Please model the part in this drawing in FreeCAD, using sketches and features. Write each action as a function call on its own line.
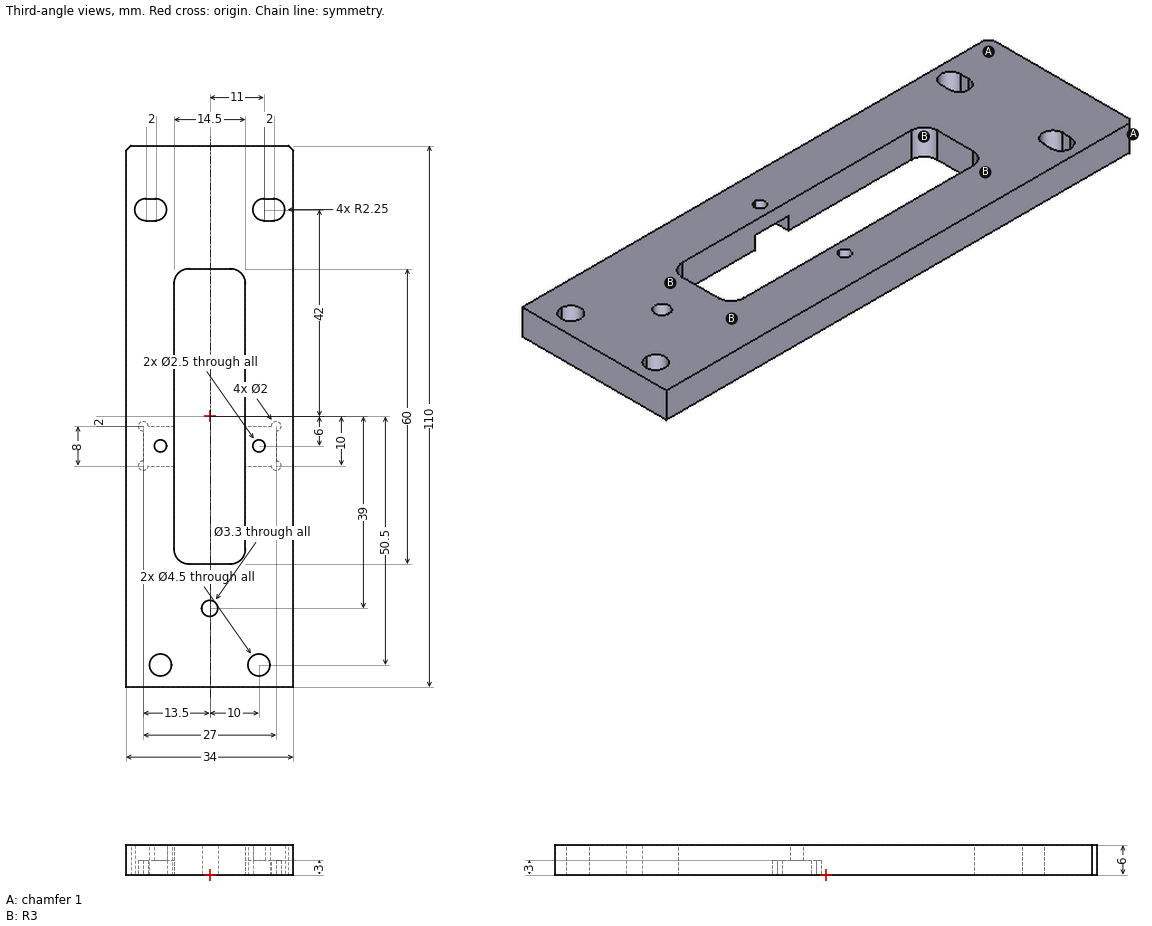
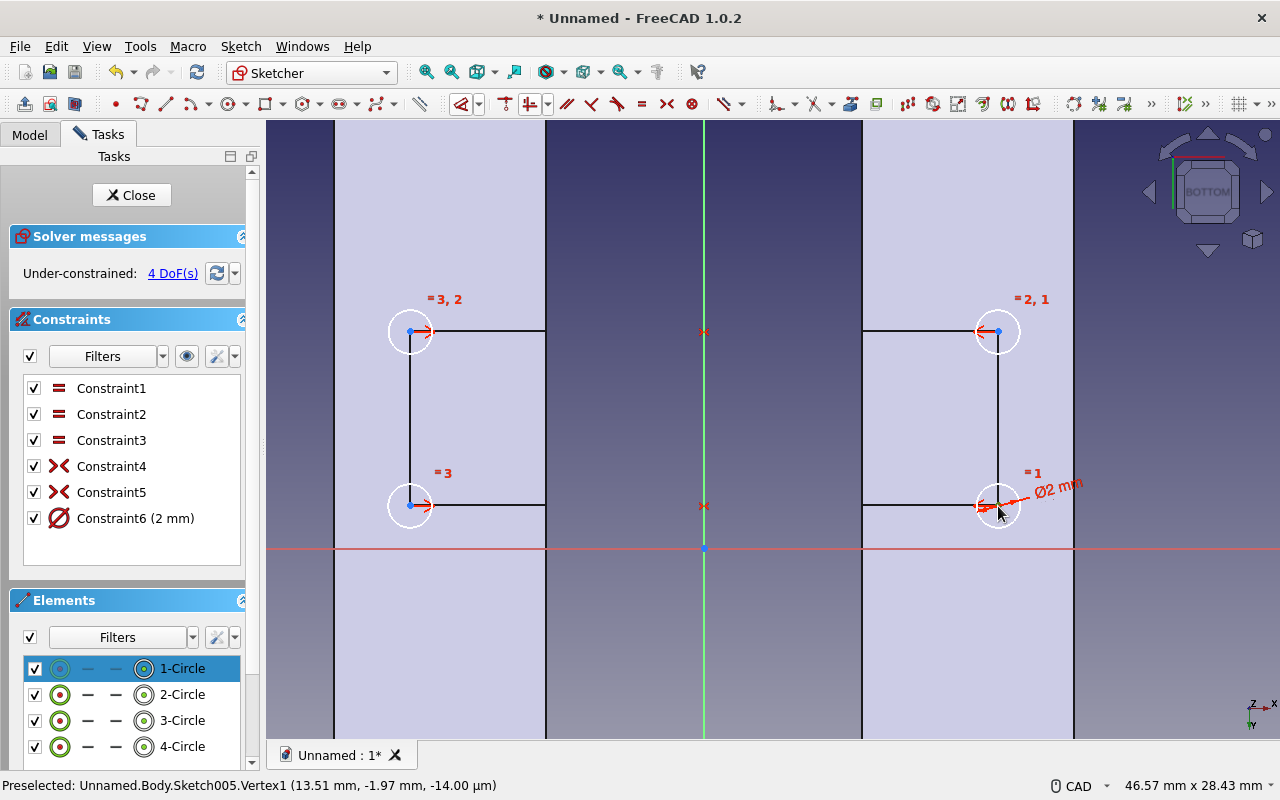
key(i)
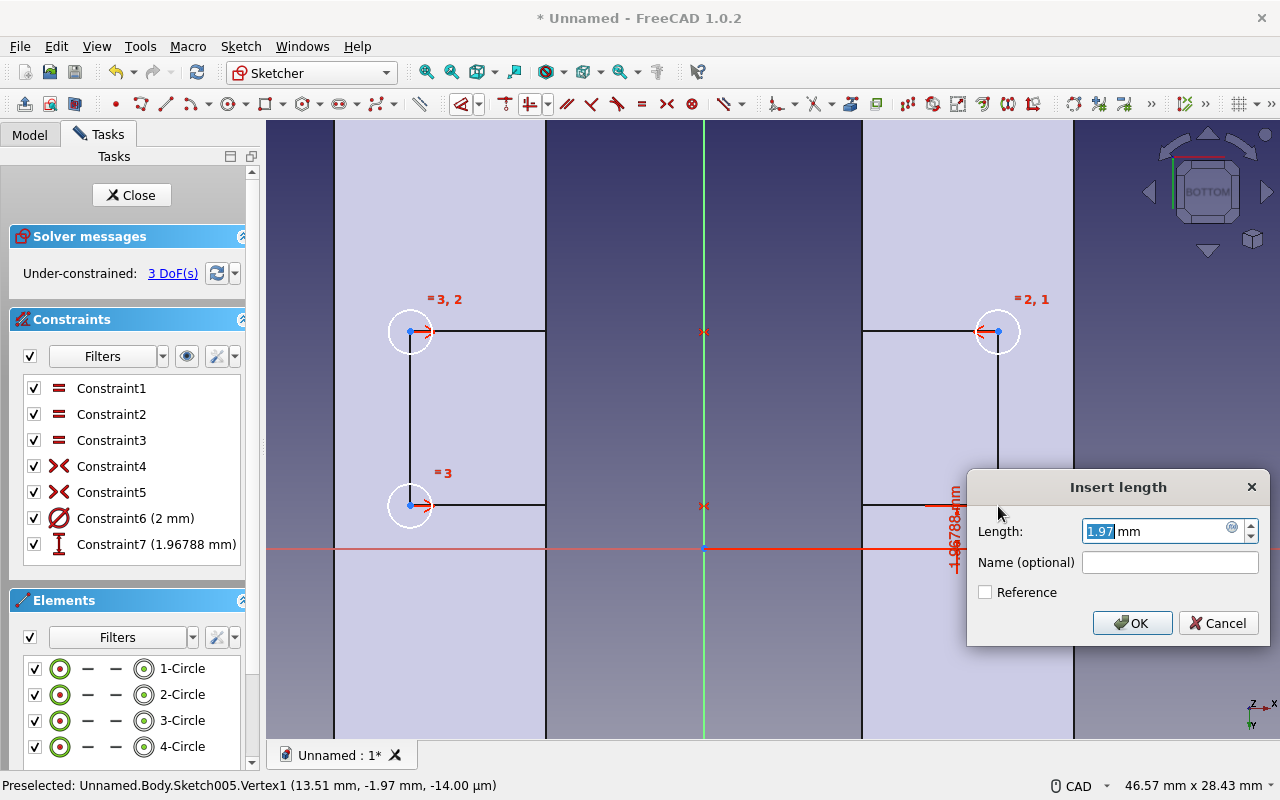
text(2)
key(Return)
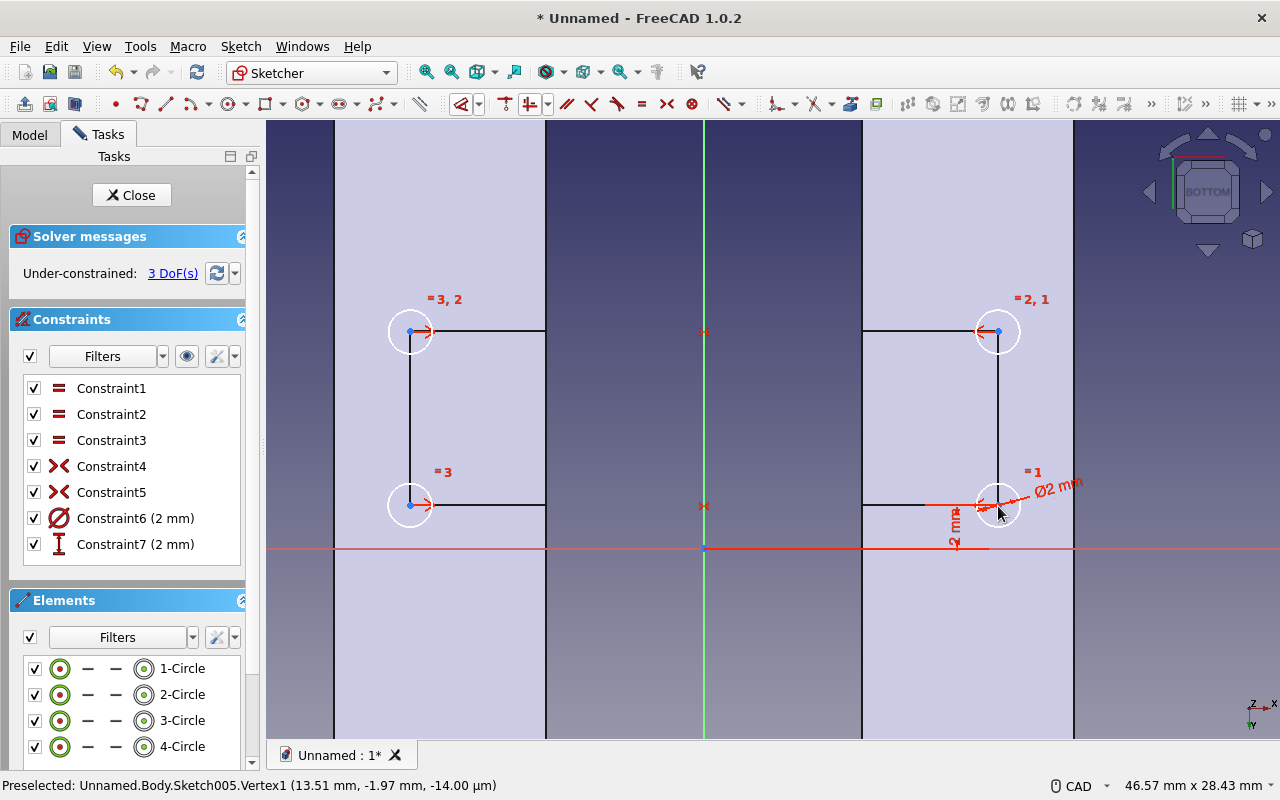
click(998, 332)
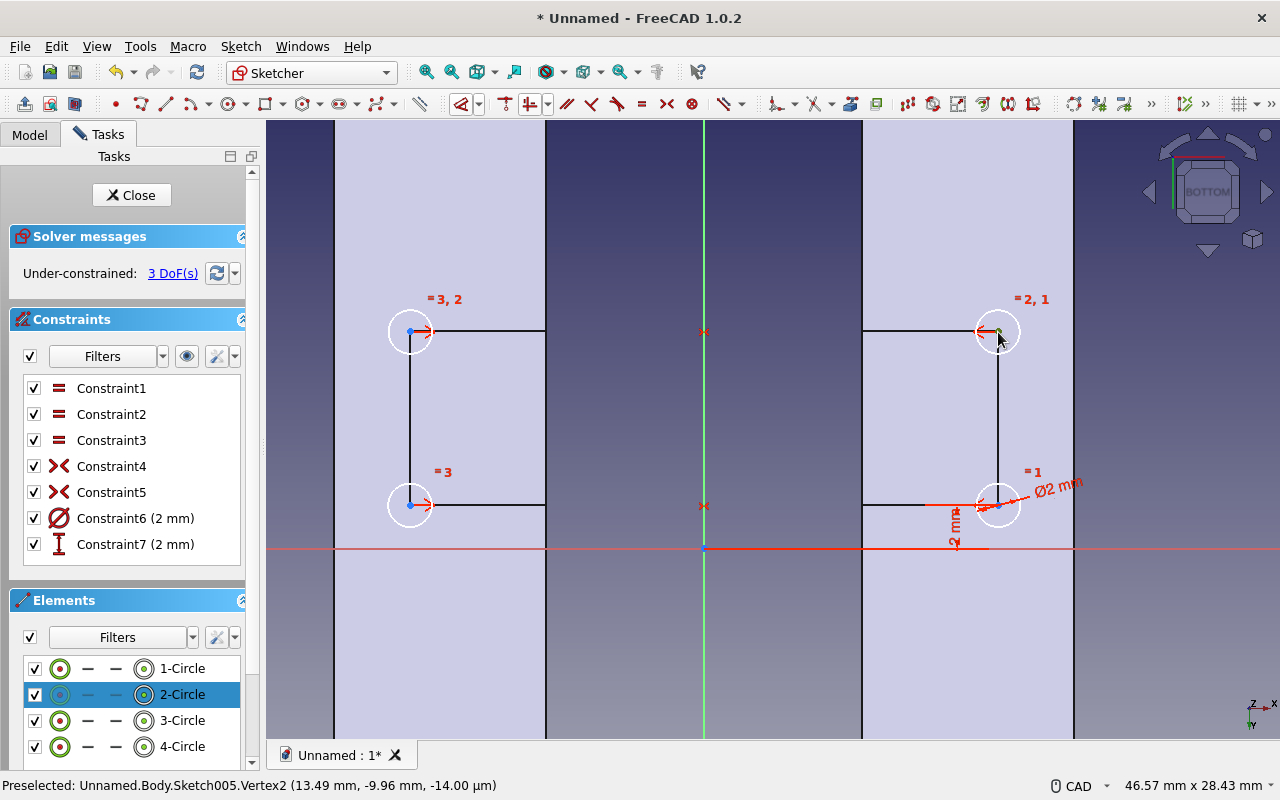
key(i)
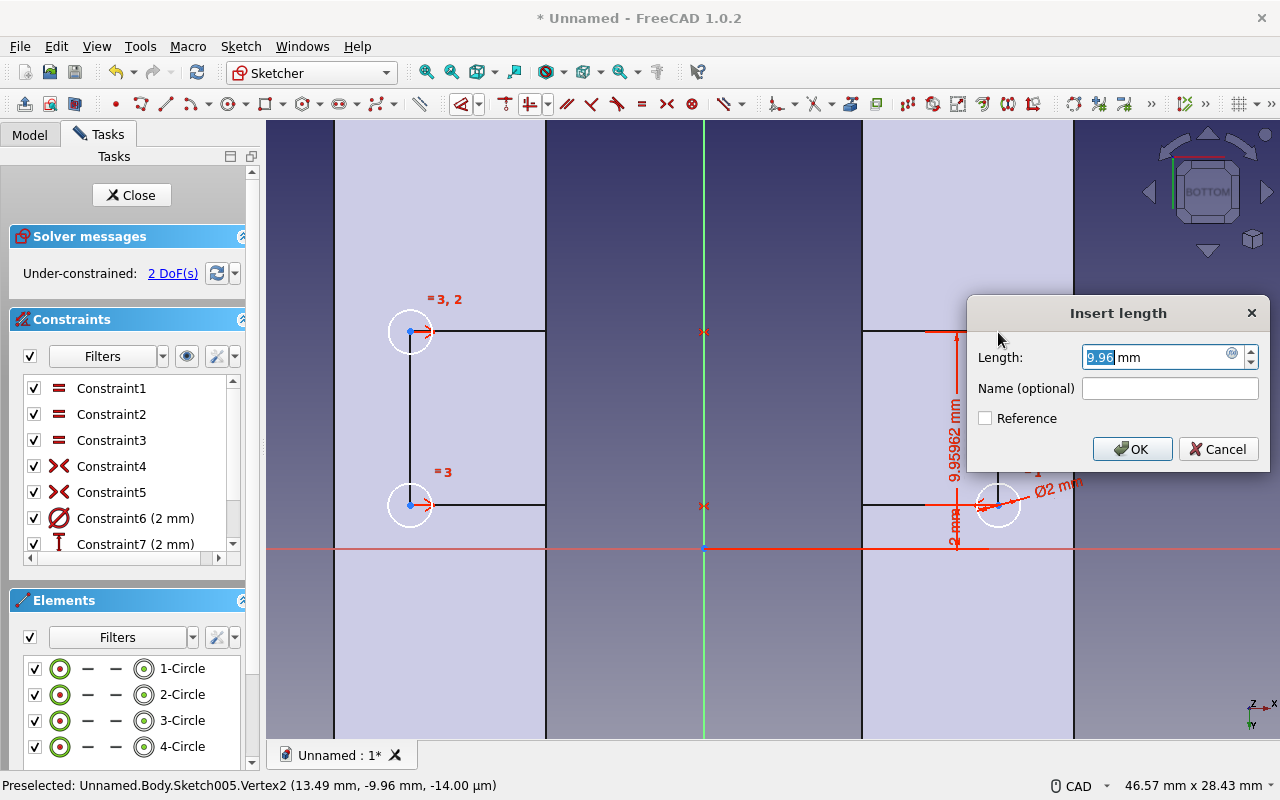
text(10)
key(Return)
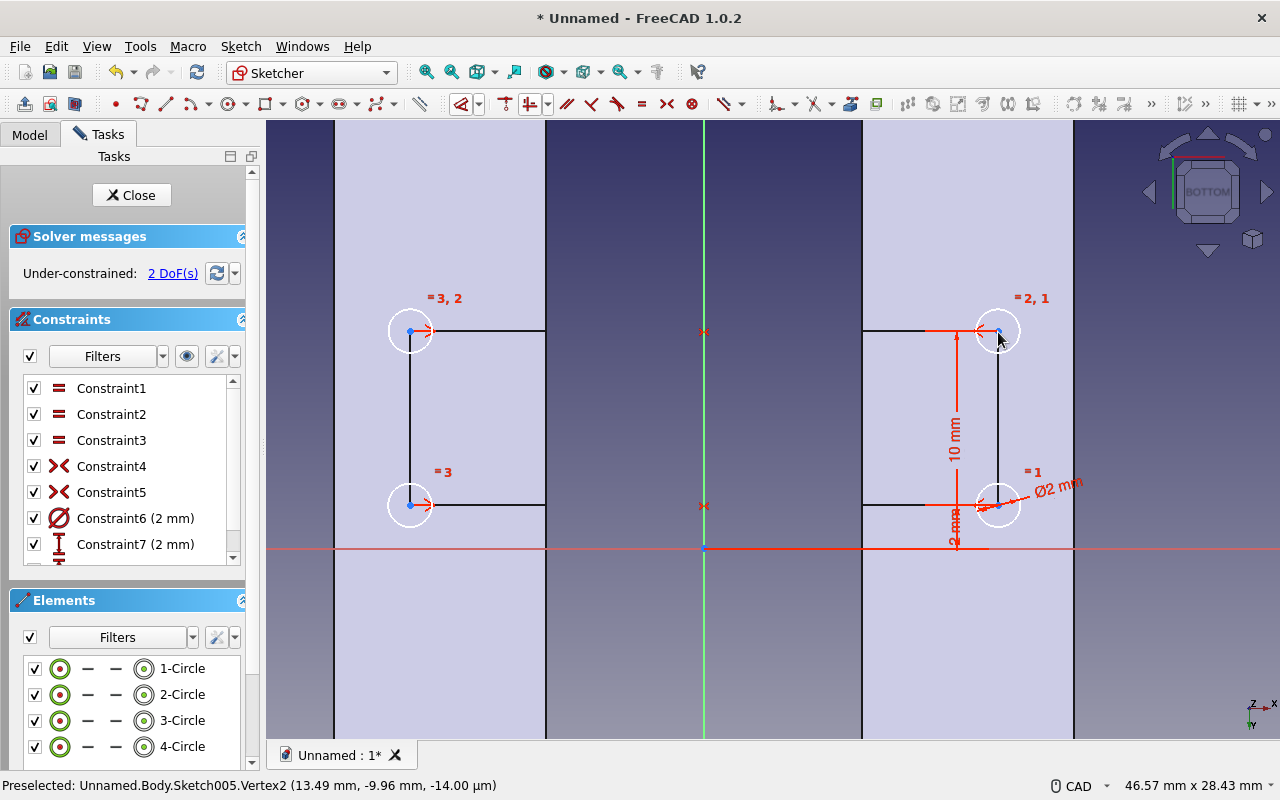
click(998, 331)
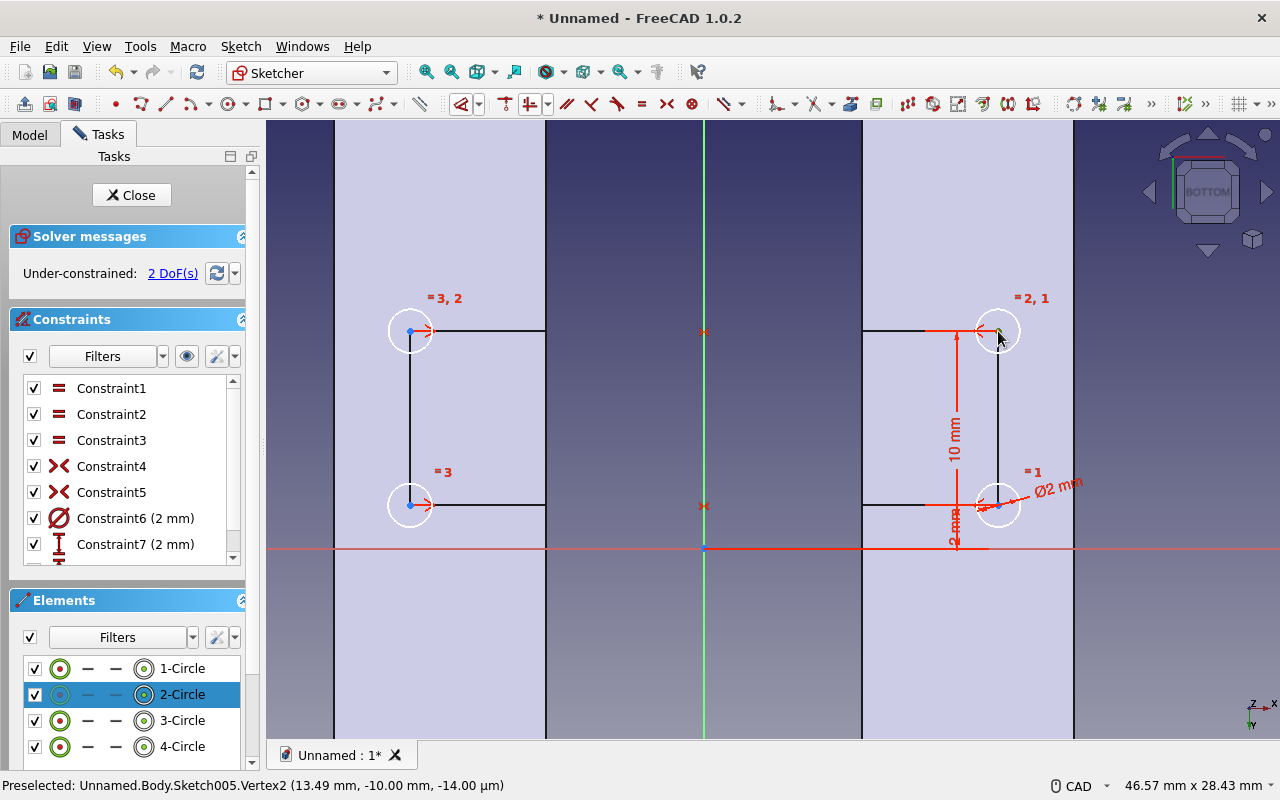
click(410, 331)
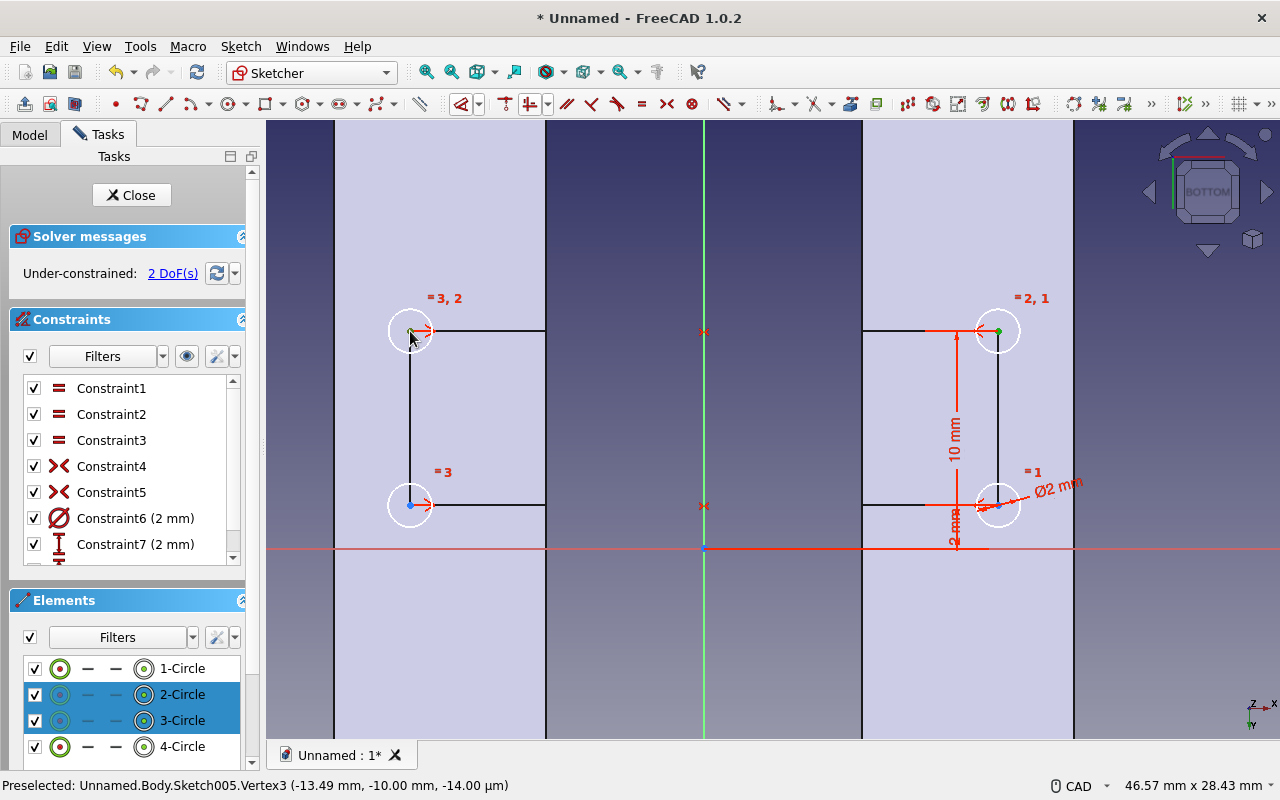
click(478, 104)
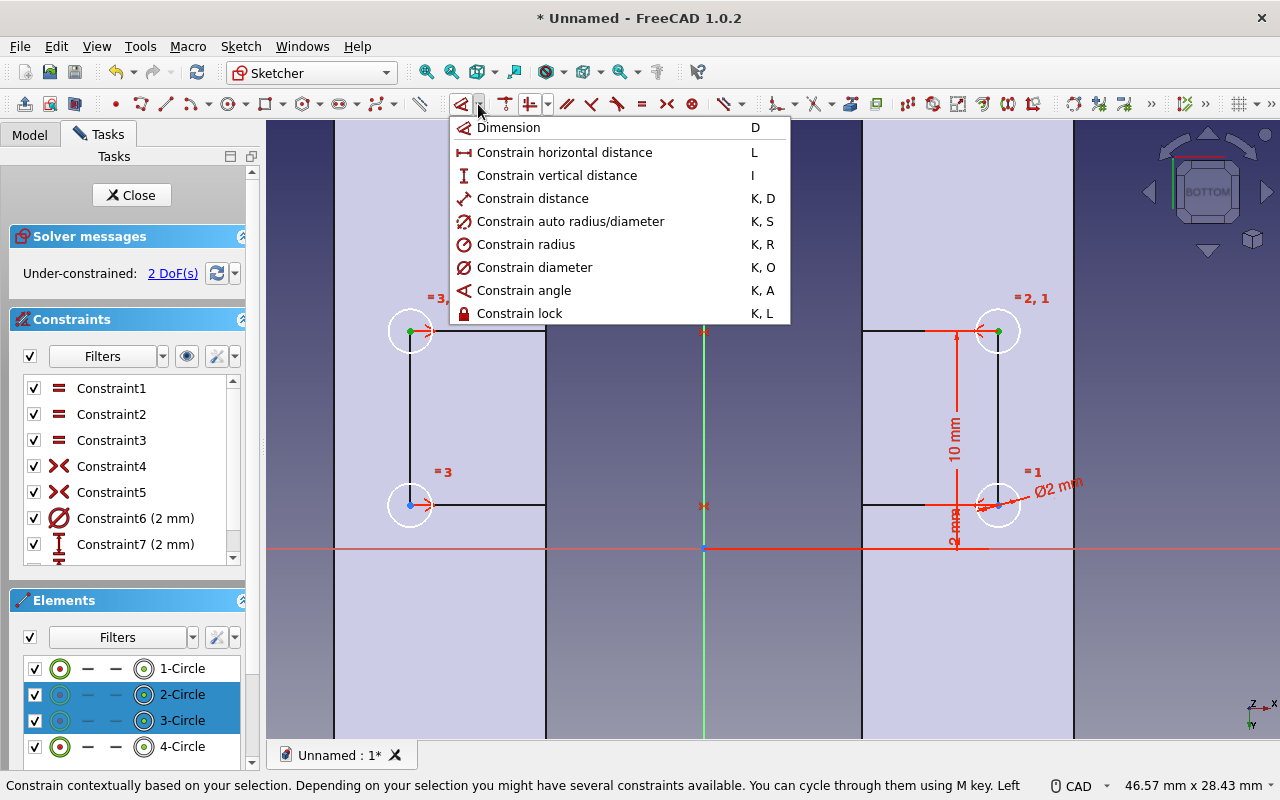
click(620, 152)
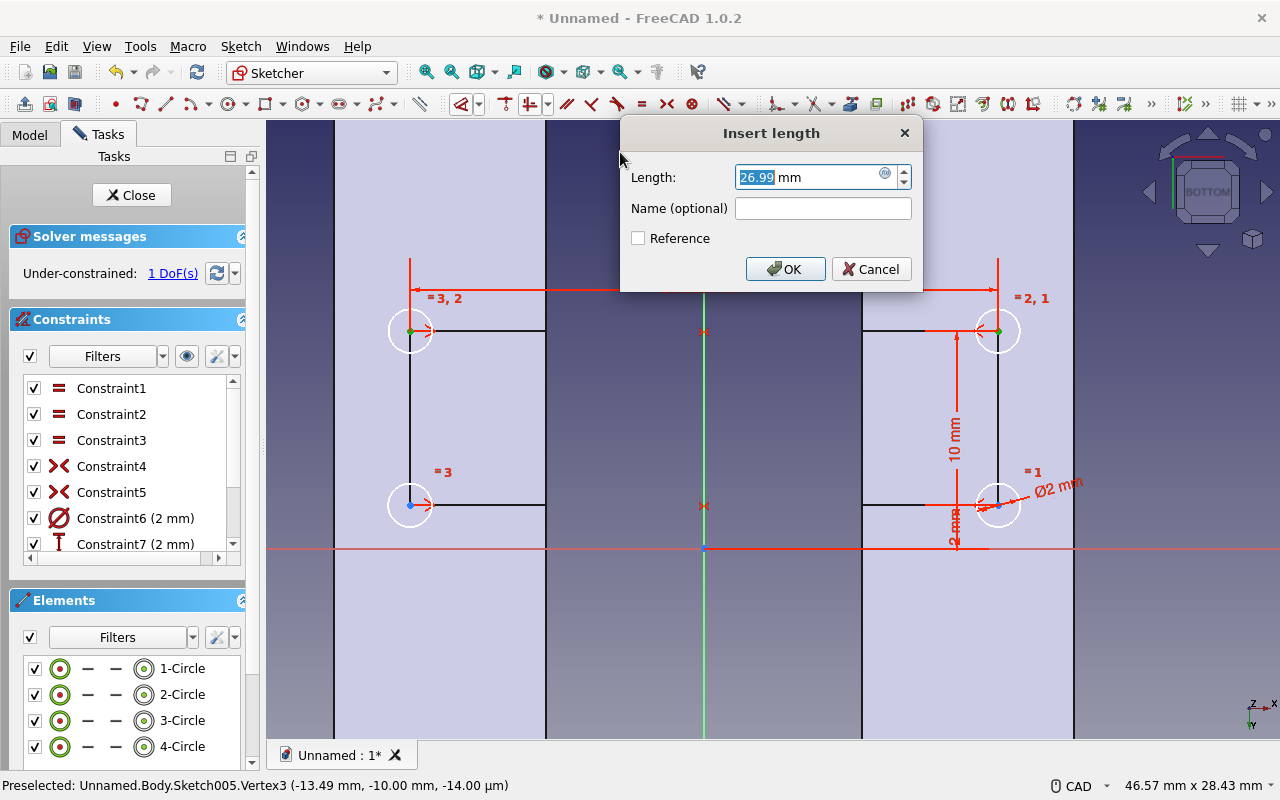
text(27)
key(Return)